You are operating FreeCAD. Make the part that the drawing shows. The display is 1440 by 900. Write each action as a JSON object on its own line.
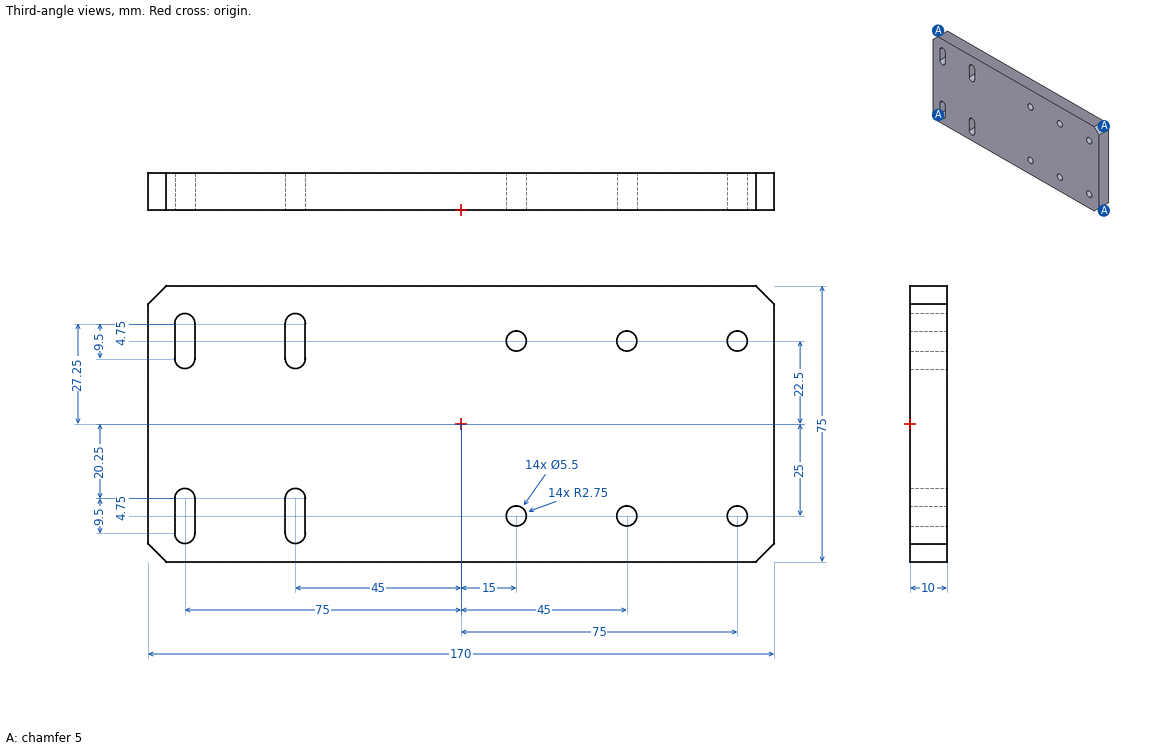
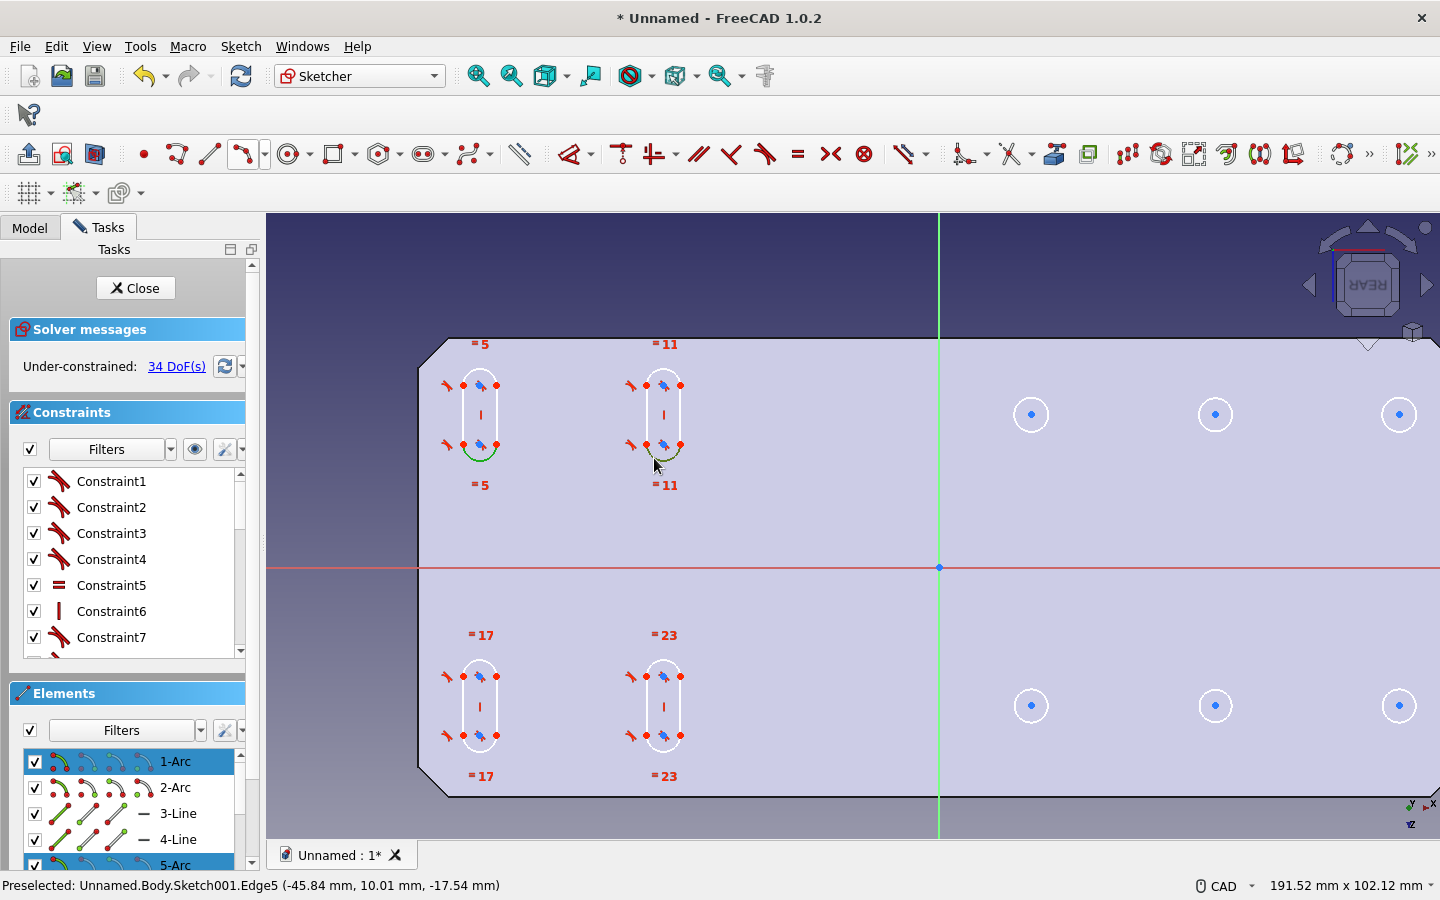
{"action": "left_click", "coordinate": [470, 749]}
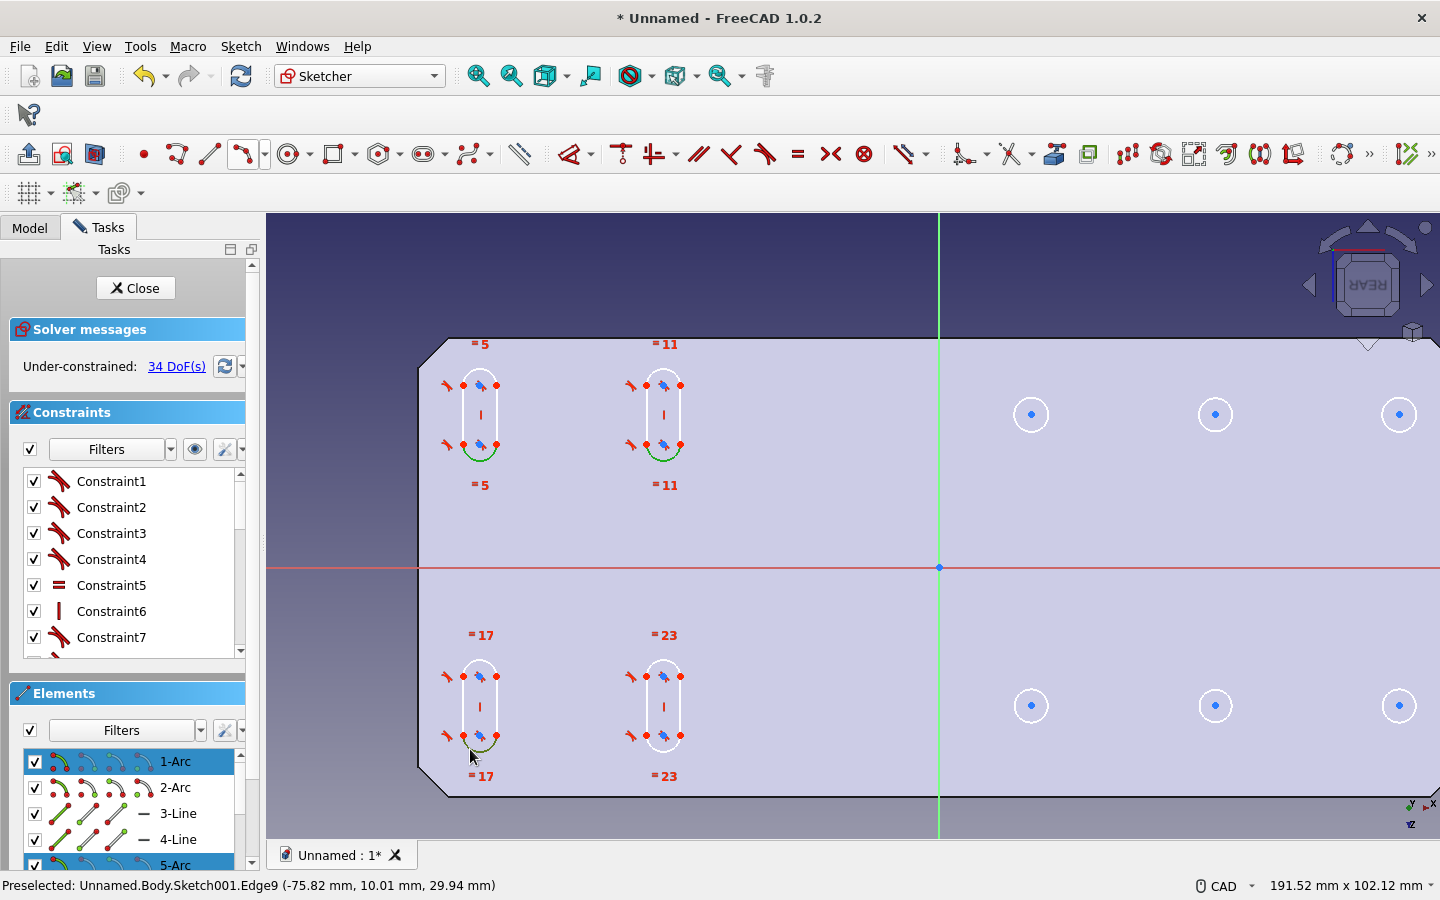
{"action": "left_click", "coordinate": [654, 749]}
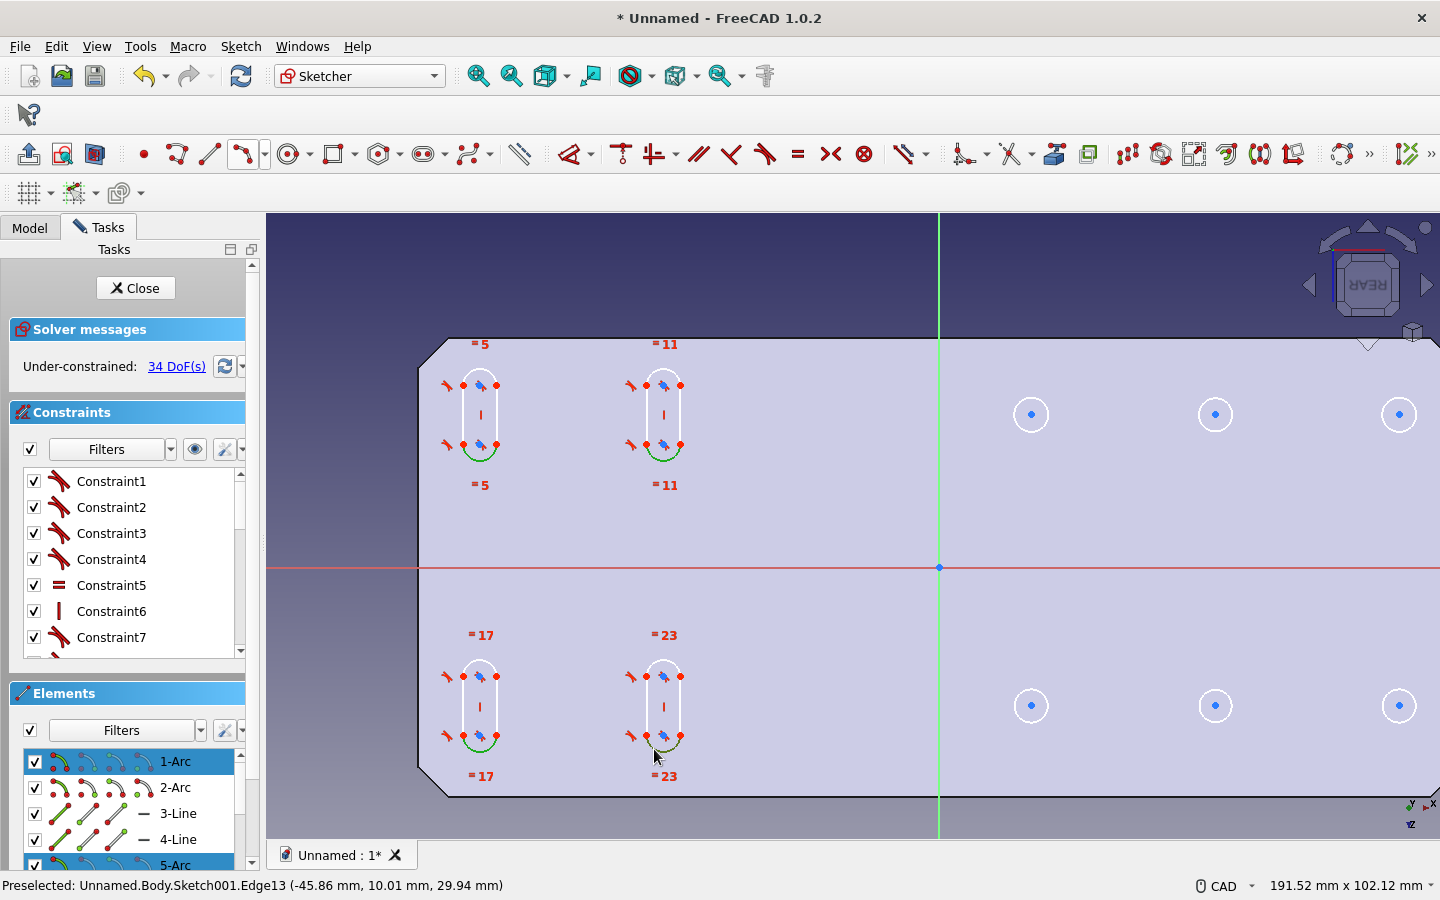
{"action": "key", "text": "e"}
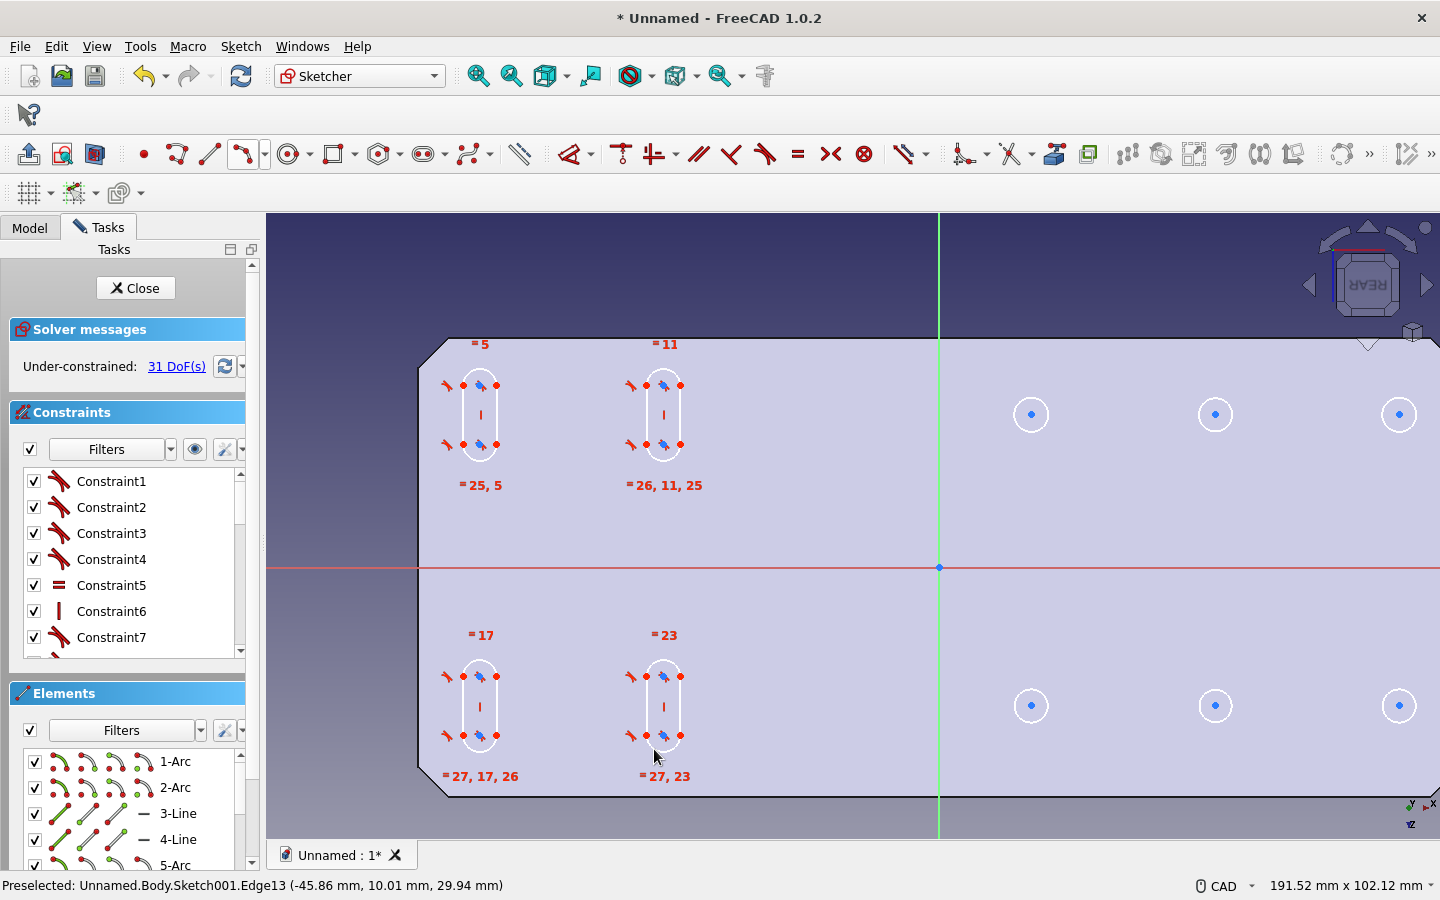
{"action": "left_click", "coordinate": [1043, 403]}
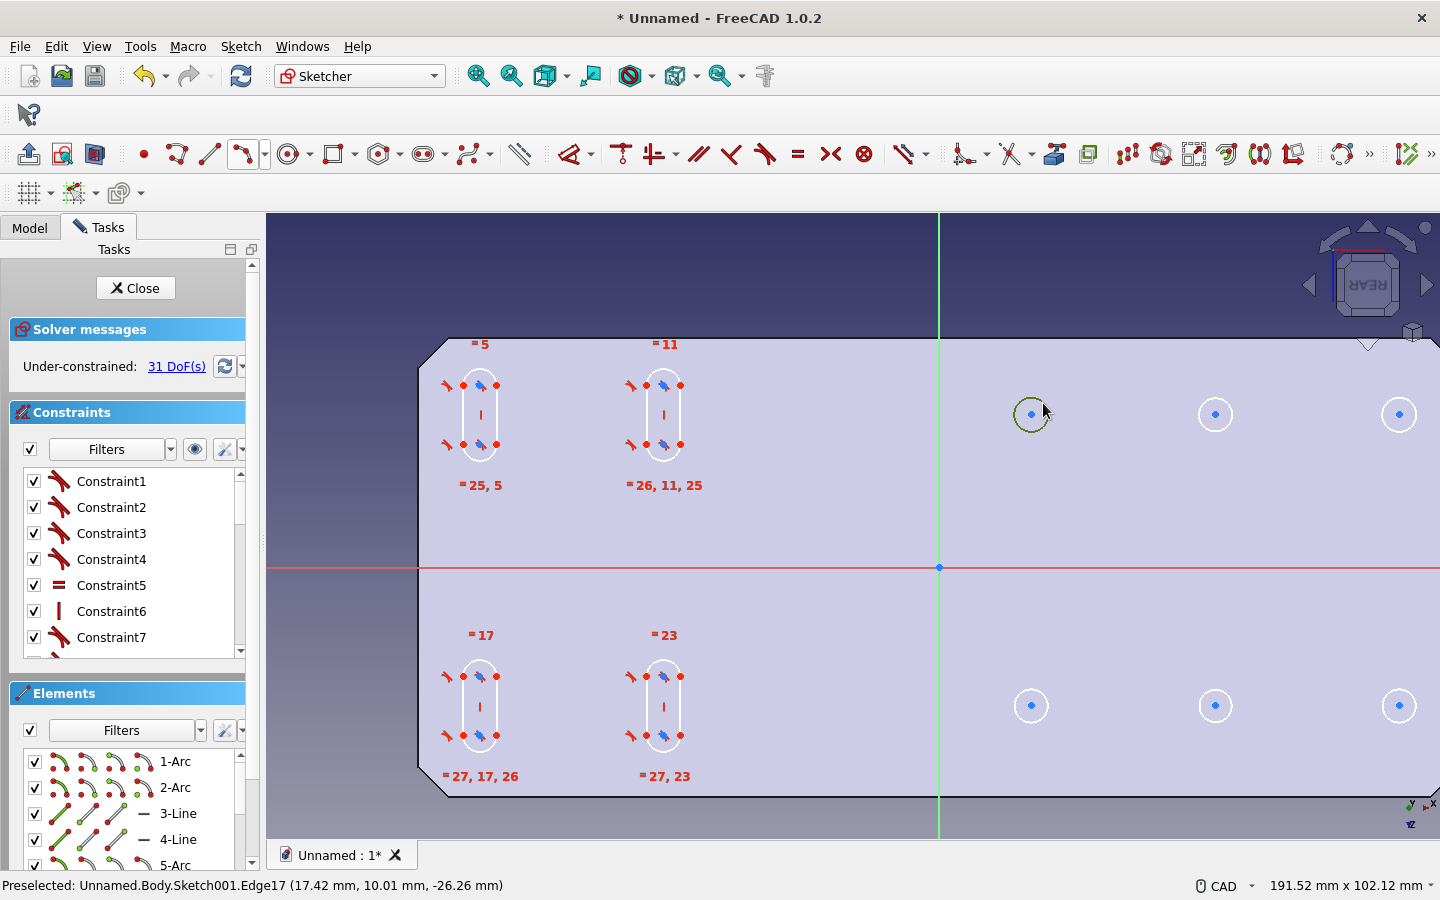
{"action": "left_click", "coordinate": [1227, 403]}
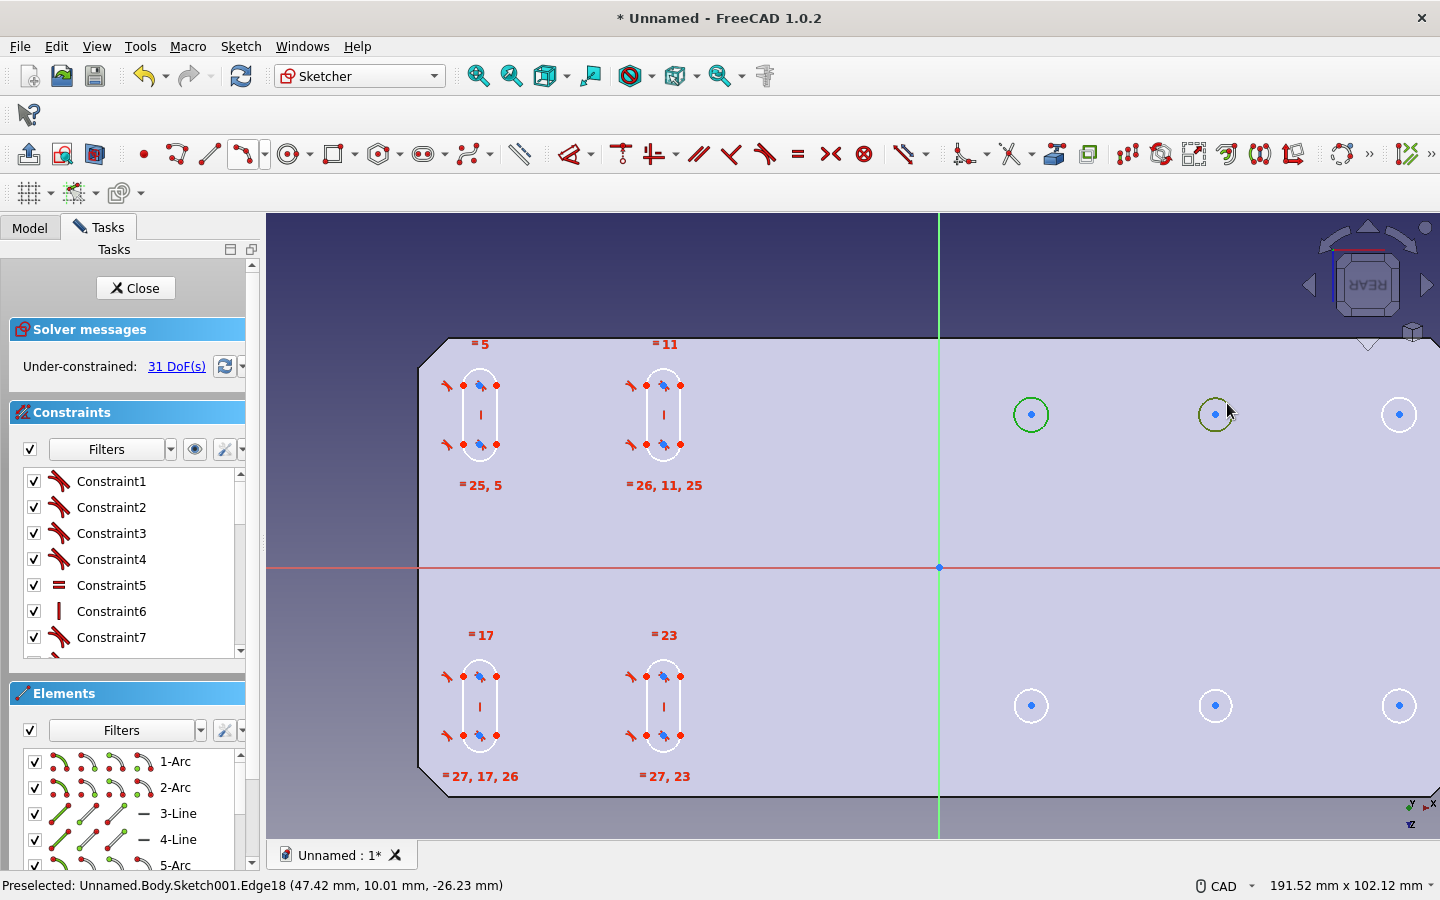
{"action": "scroll", "coordinate": [469, 457], "scroll_direction": "down", "scroll_amount": 2}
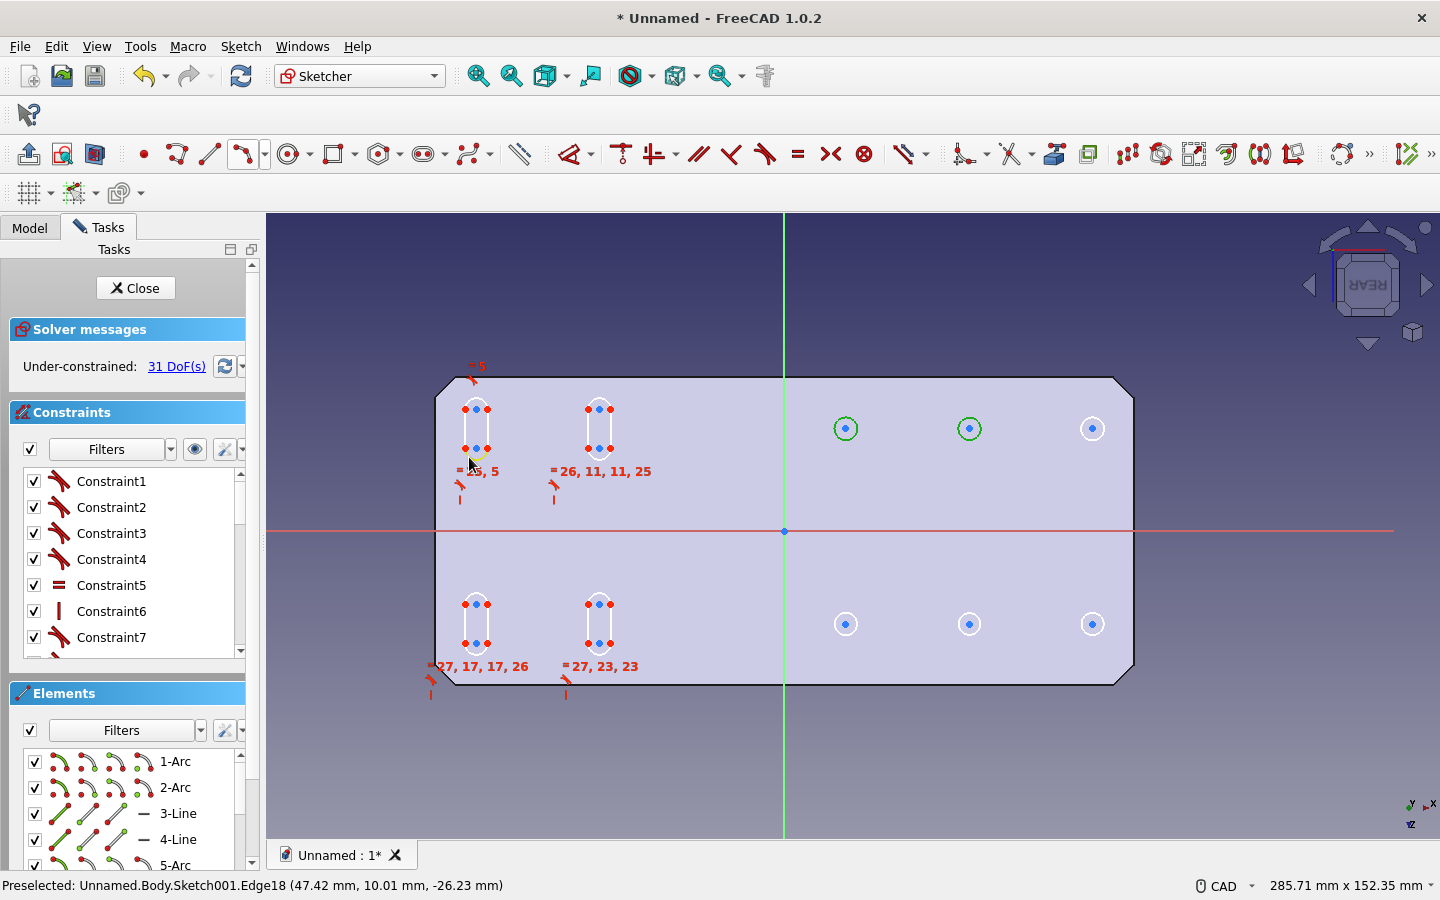
{"action": "left_click", "coordinate": [1101, 421]}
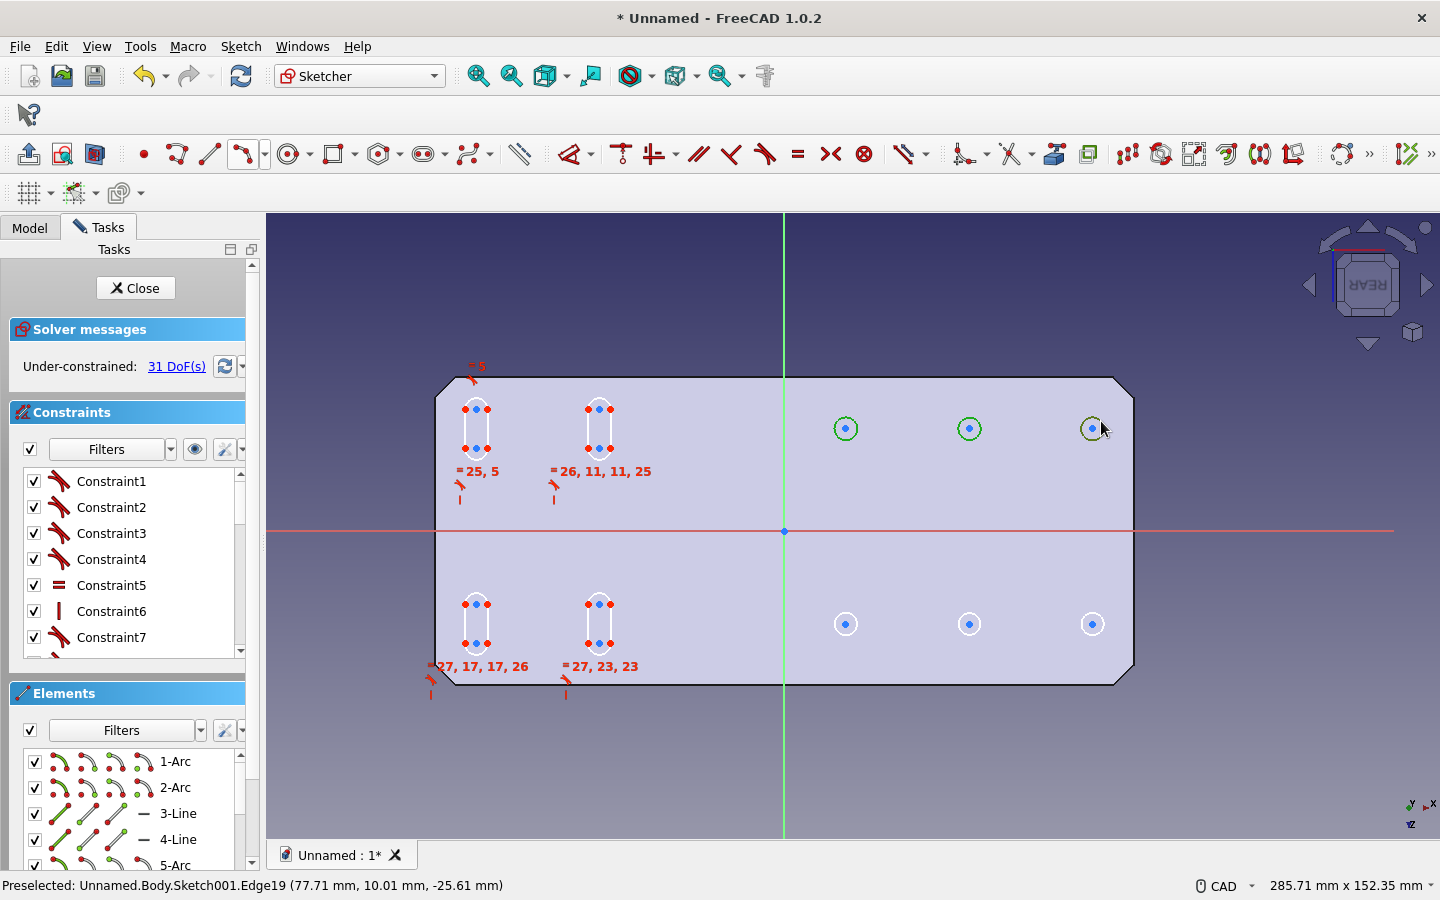
{"action": "scroll", "coordinate": [854, 616], "scroll_direction": "up", "scroll_amount": 2}